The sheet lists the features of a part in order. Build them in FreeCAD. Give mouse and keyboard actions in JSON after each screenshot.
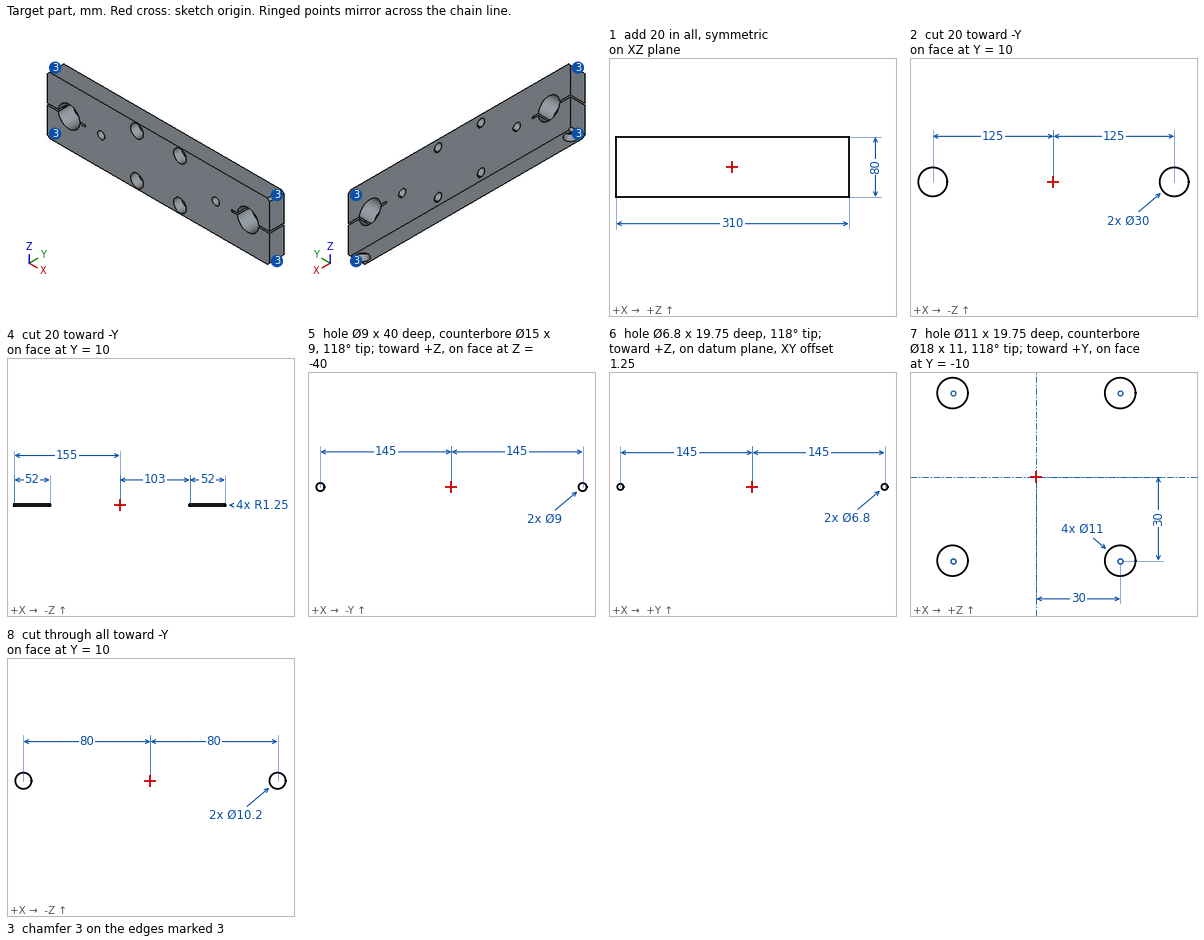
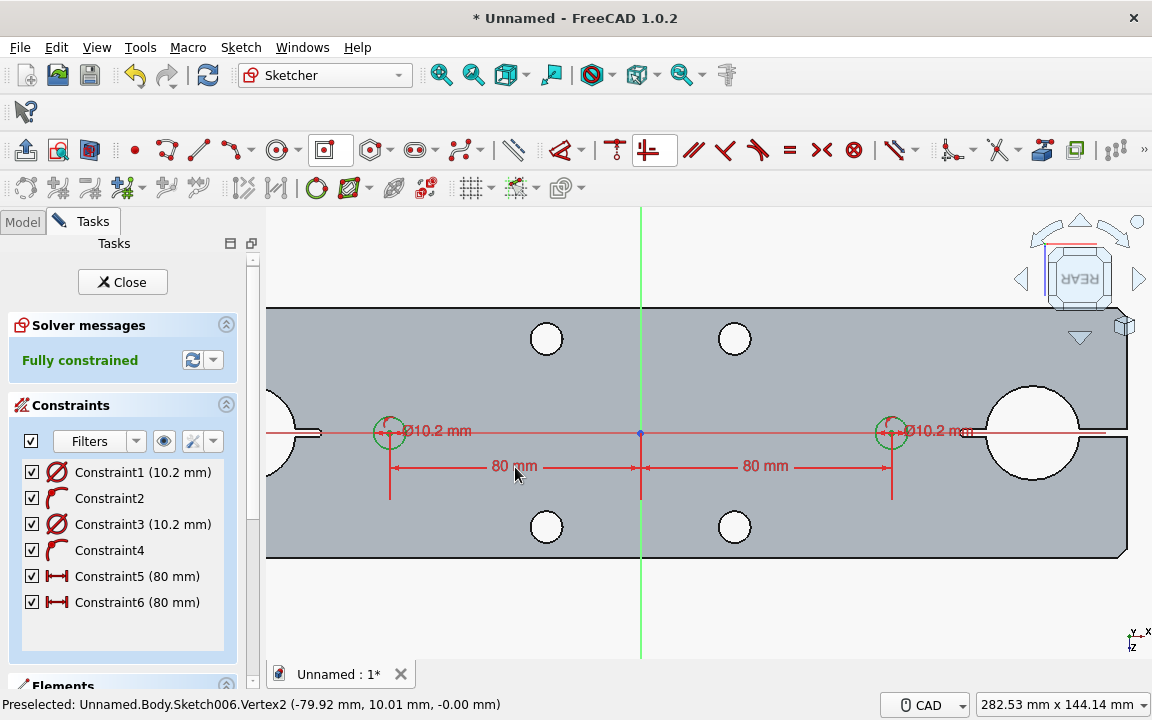
{"action": "left_click", "coordinate": [123, 282]}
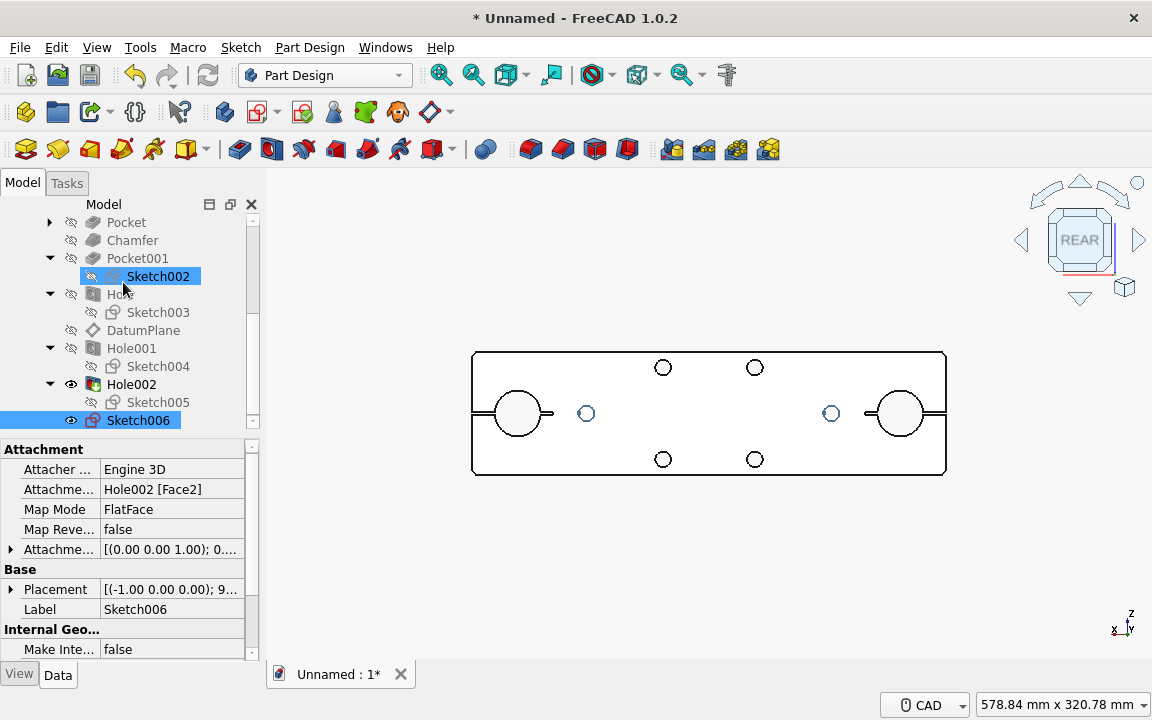
{"action": "left_click", "coordinate": [240, 150]}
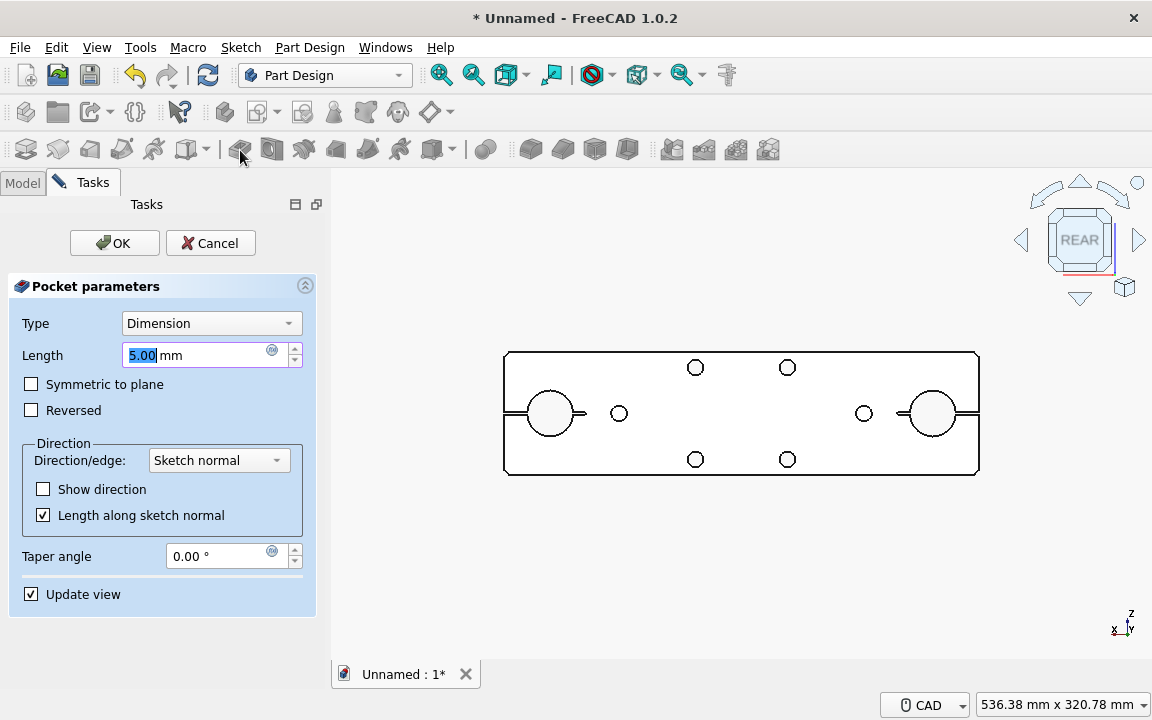
{"action": "left_click", "coordinate": [212, 324]}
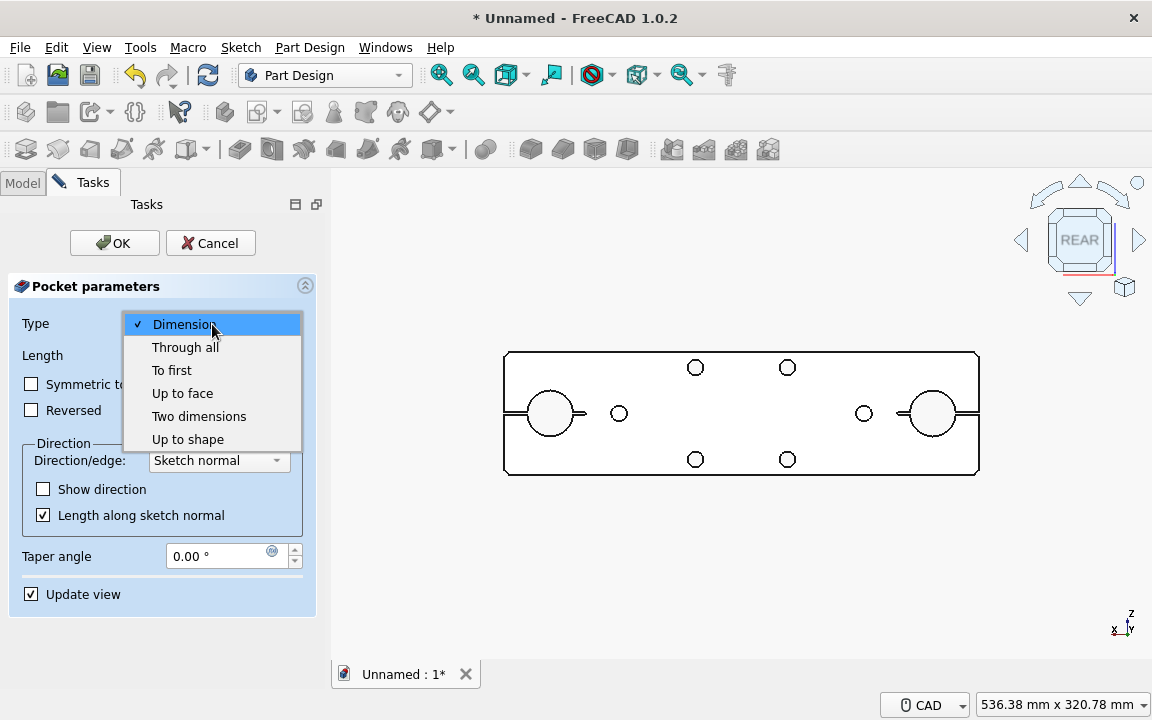
{"action": "left_click", "coordinate": [212, 348]}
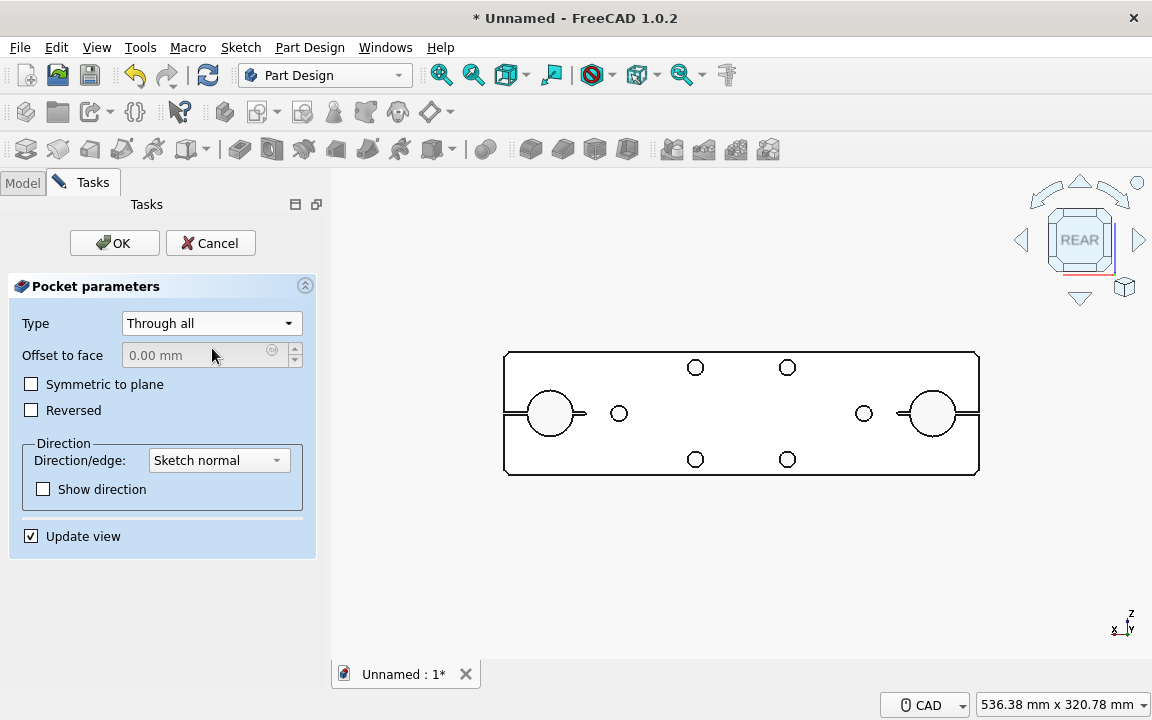
{"action": "left_click", "coordinate": [115, 243]}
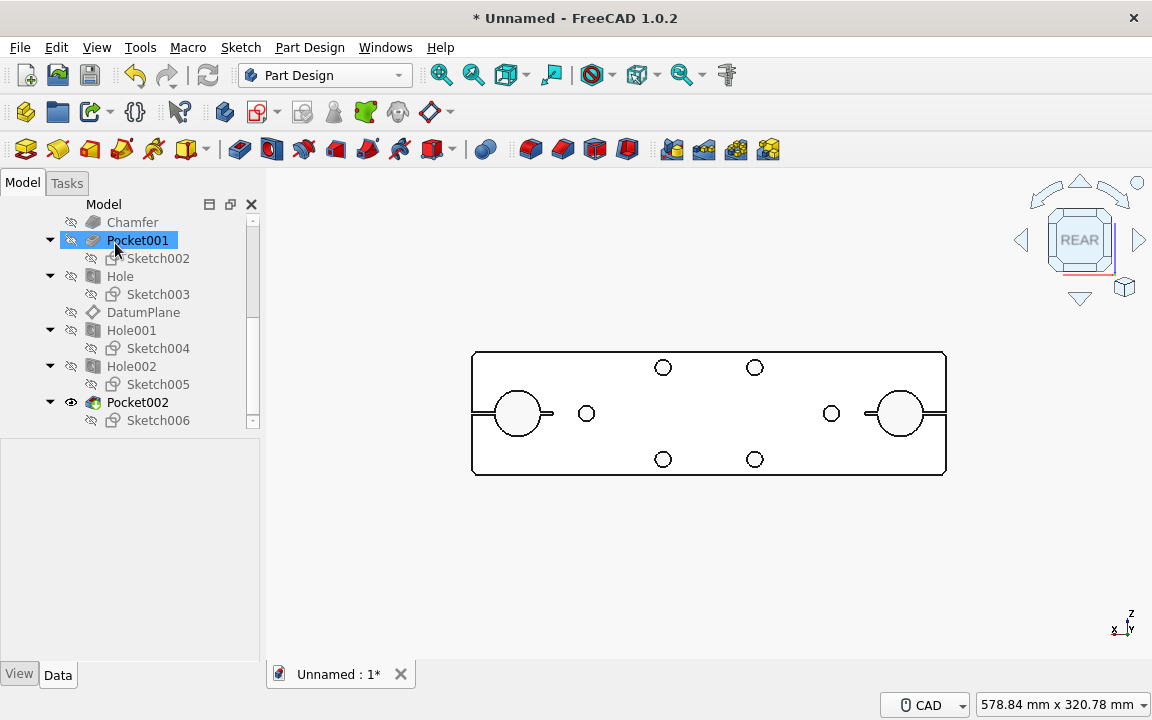
{"action": "key", "text": "0"}